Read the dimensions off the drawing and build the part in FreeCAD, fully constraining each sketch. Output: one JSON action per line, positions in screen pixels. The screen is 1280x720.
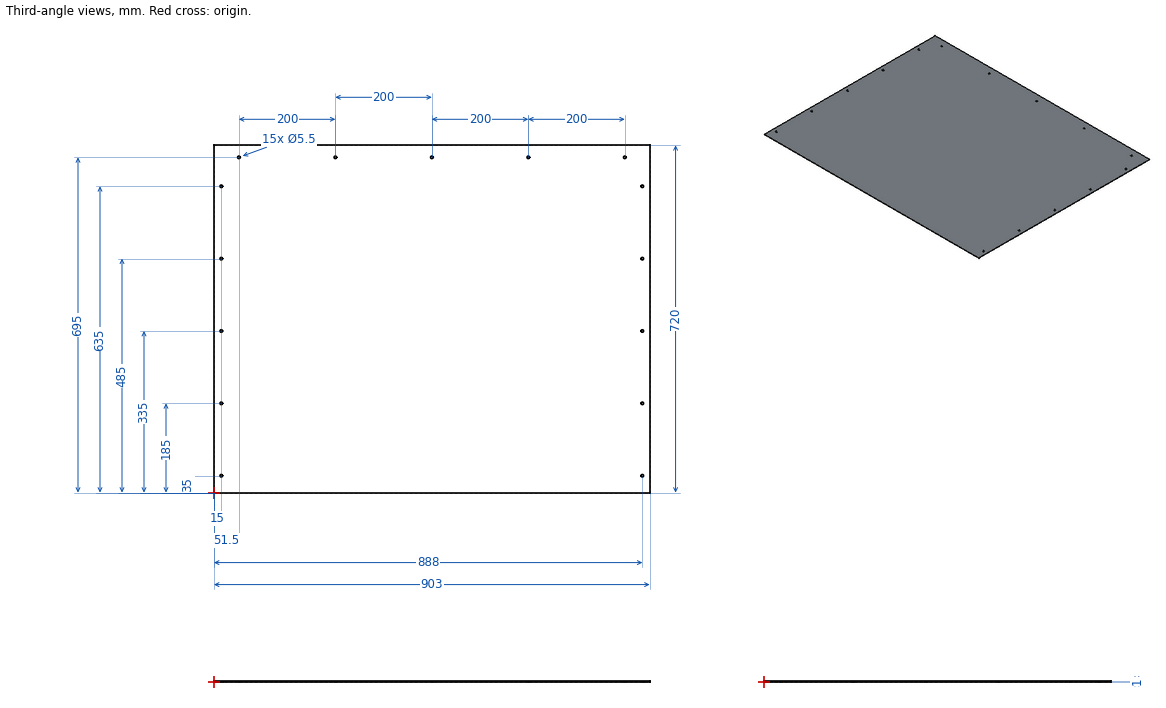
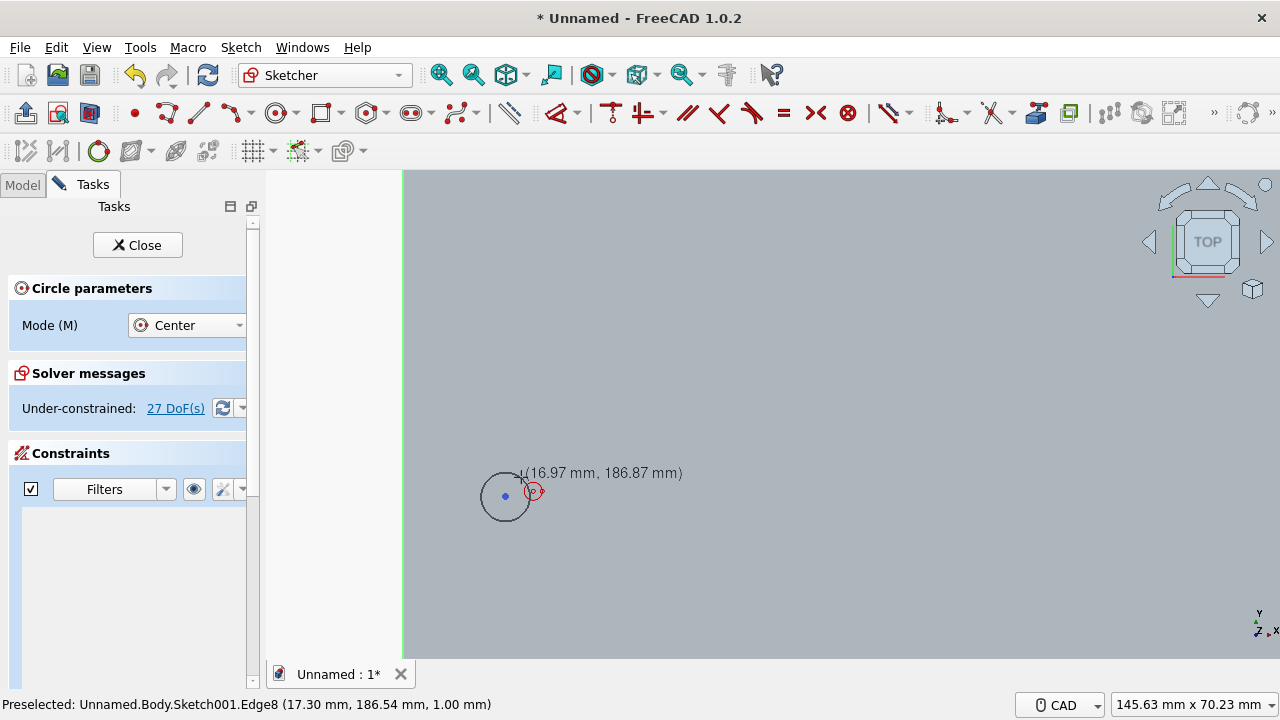
{"action": "scroll", "coordinate": [523, 483], "scroll_direction": "down", "scroll_amount": 14}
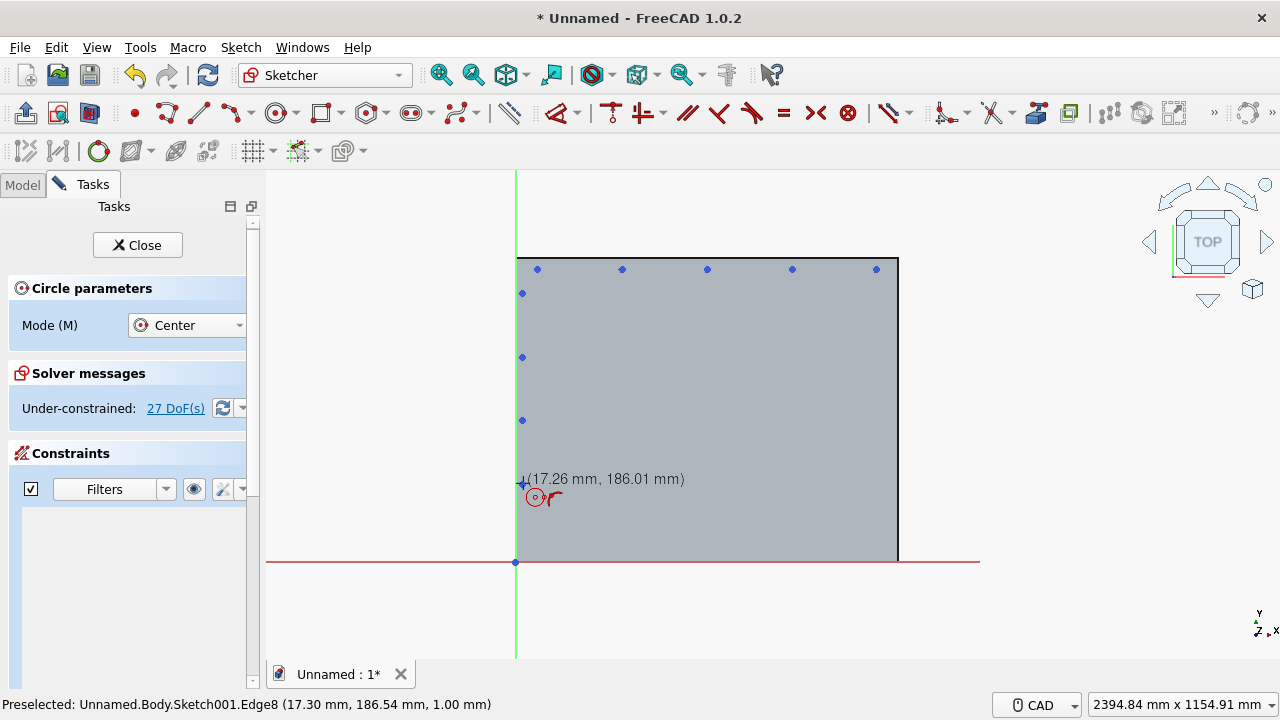
{"action": "scroll", "coordinate": [522, 548], "scroll_direction": "up", "scroll_amount": 15}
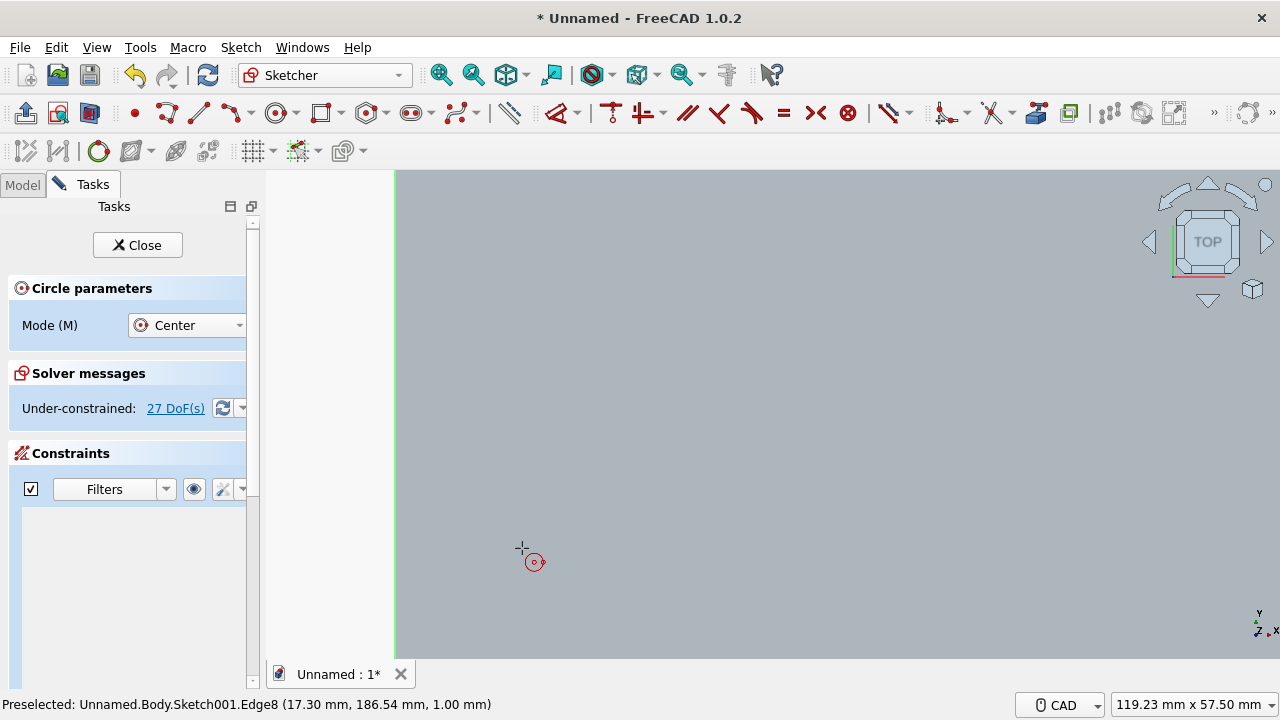
{"action": "scroll", "coordinate": [522, 549], "scroll_direction": "down", "scroll_amount": 15}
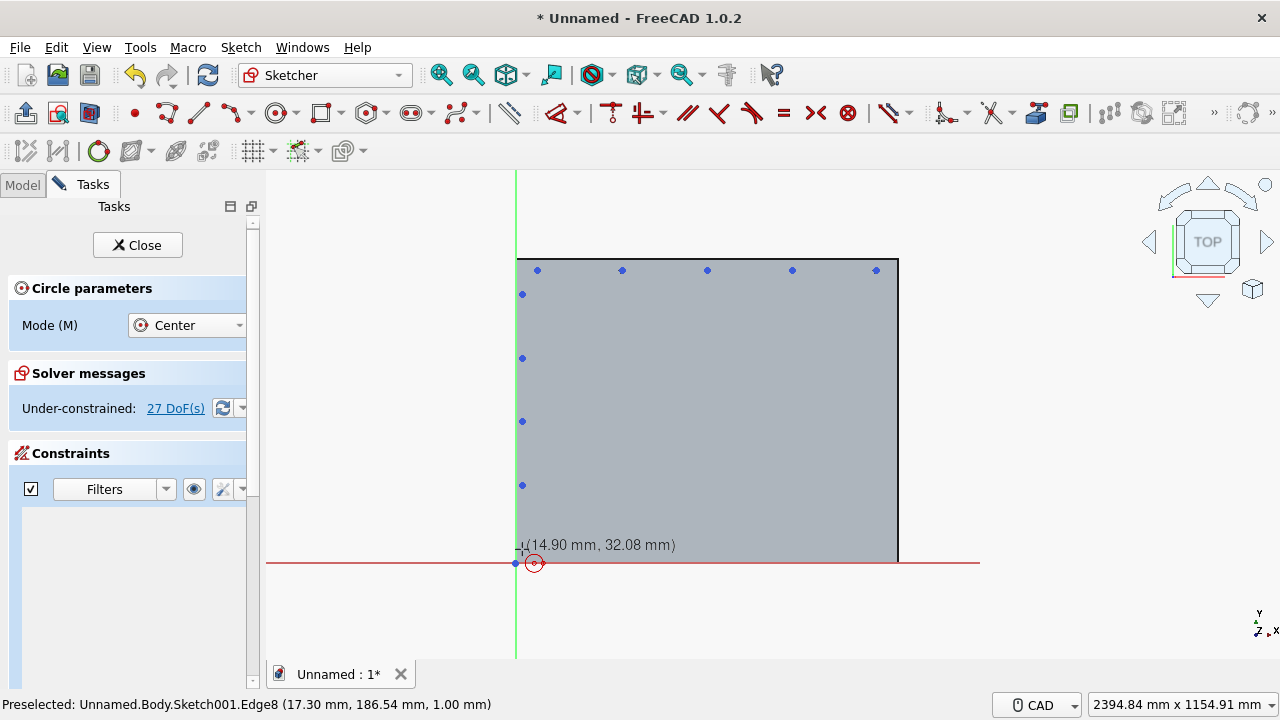
{"action": "scroll", "coordinate": [522, 549], "scroll_direction": "up", "scroll_amount": 5}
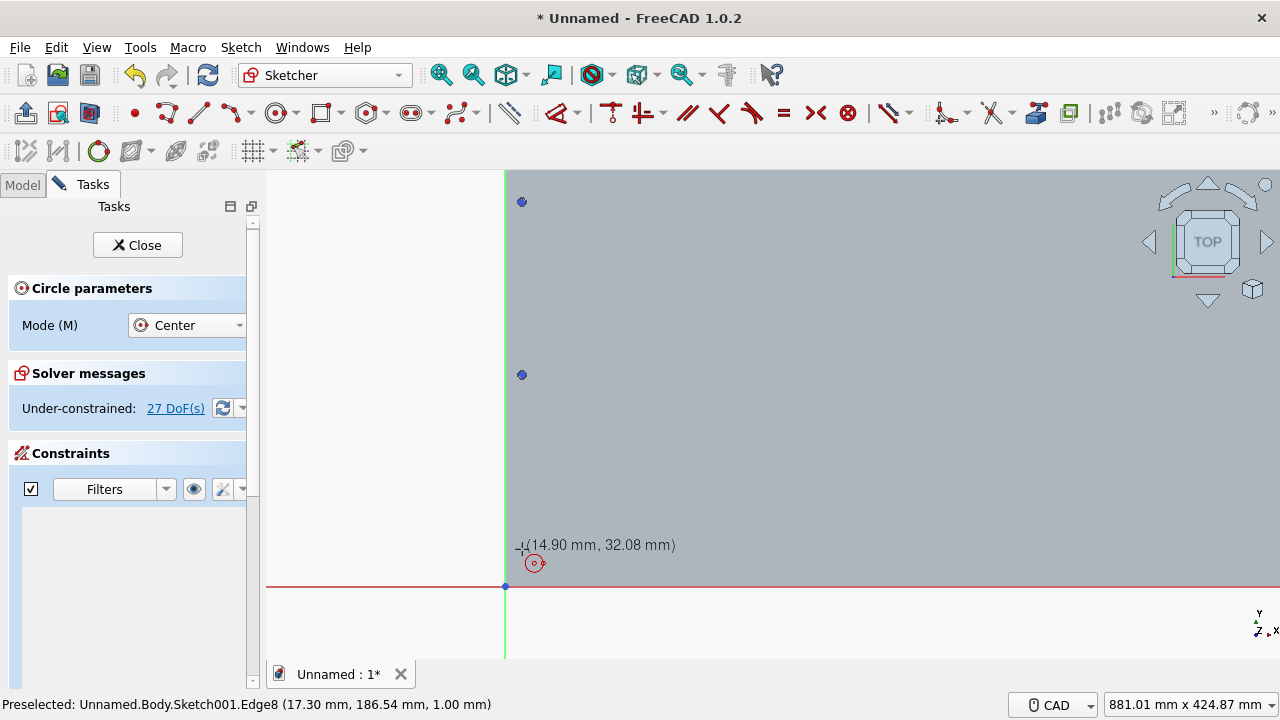
{"action": "left_click", "coordinate": [522, 546]}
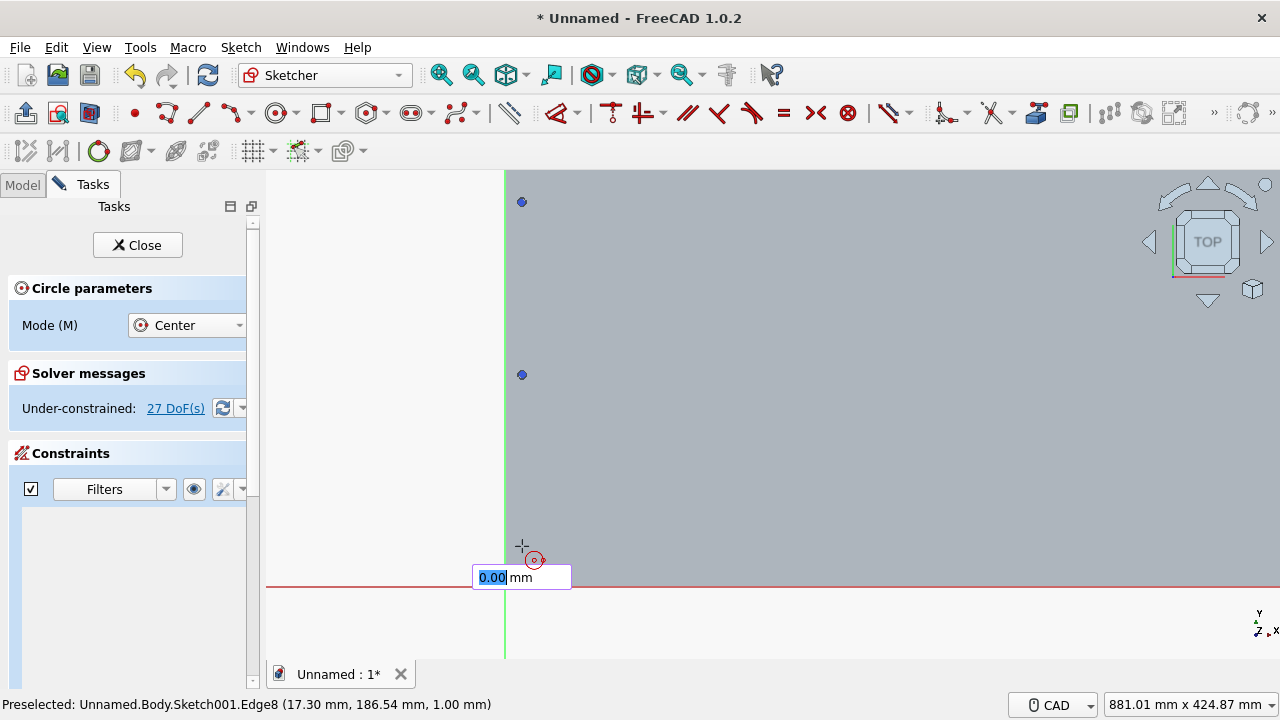
{"action": "scroll", "coordinate": [525, 544], "scroll_direction": "up", "scroll_amount": 9}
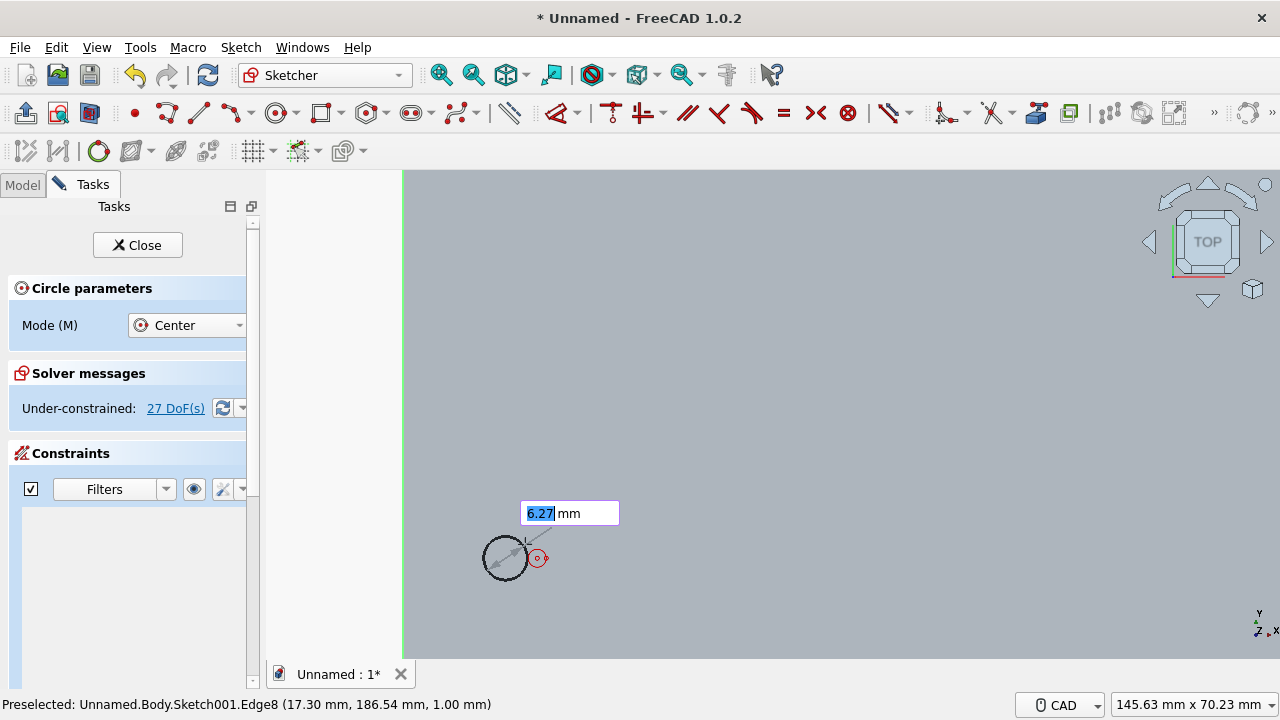
{"action": "left_click", "coordinate": [521, 541]}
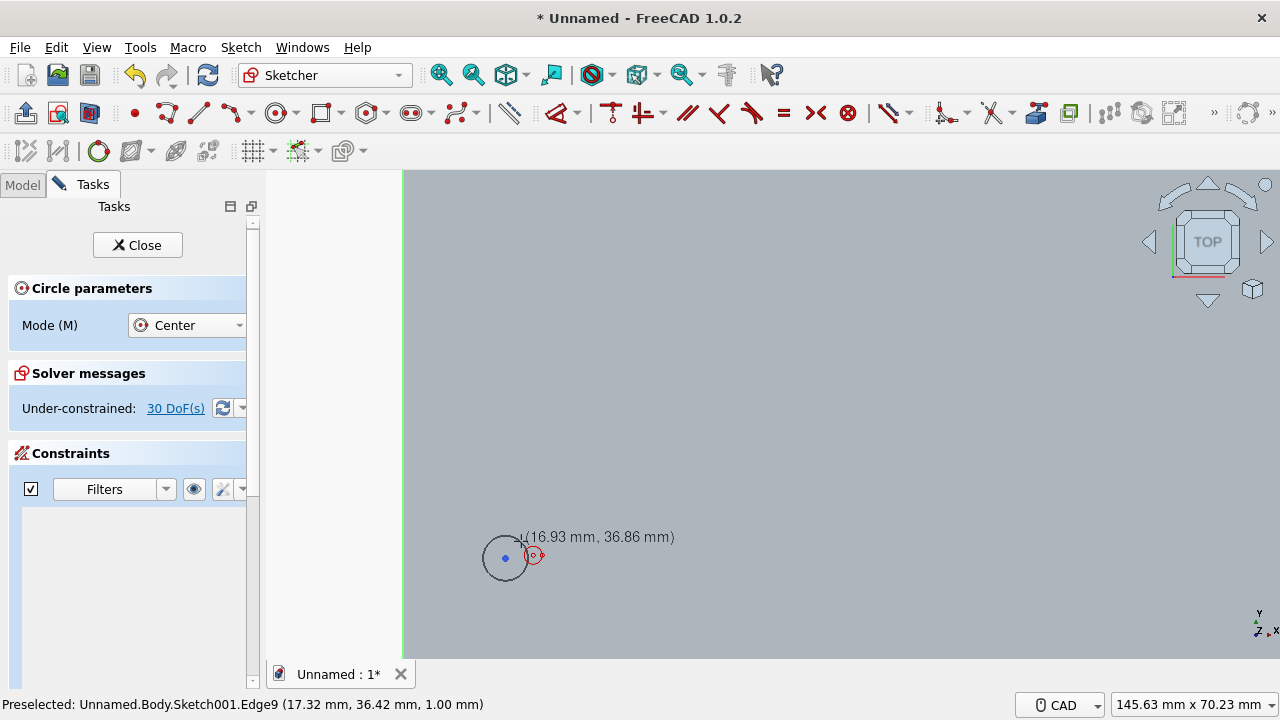
{"action": "scroll", "coordinate": [523, 547], "scroll_direction": "down", "scroll_amount": 14}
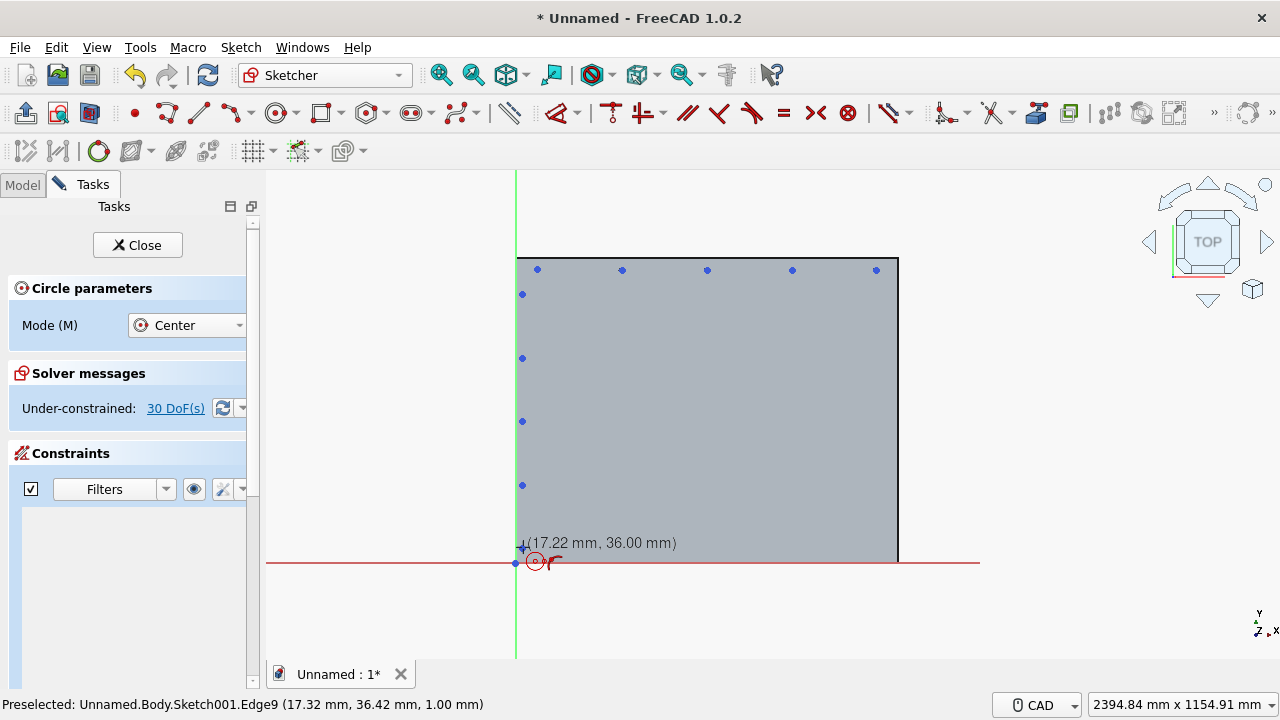
{"action": "scroll", "coordinate": [892, 548], "scroll_direction": "up", "scroll_amount": 15}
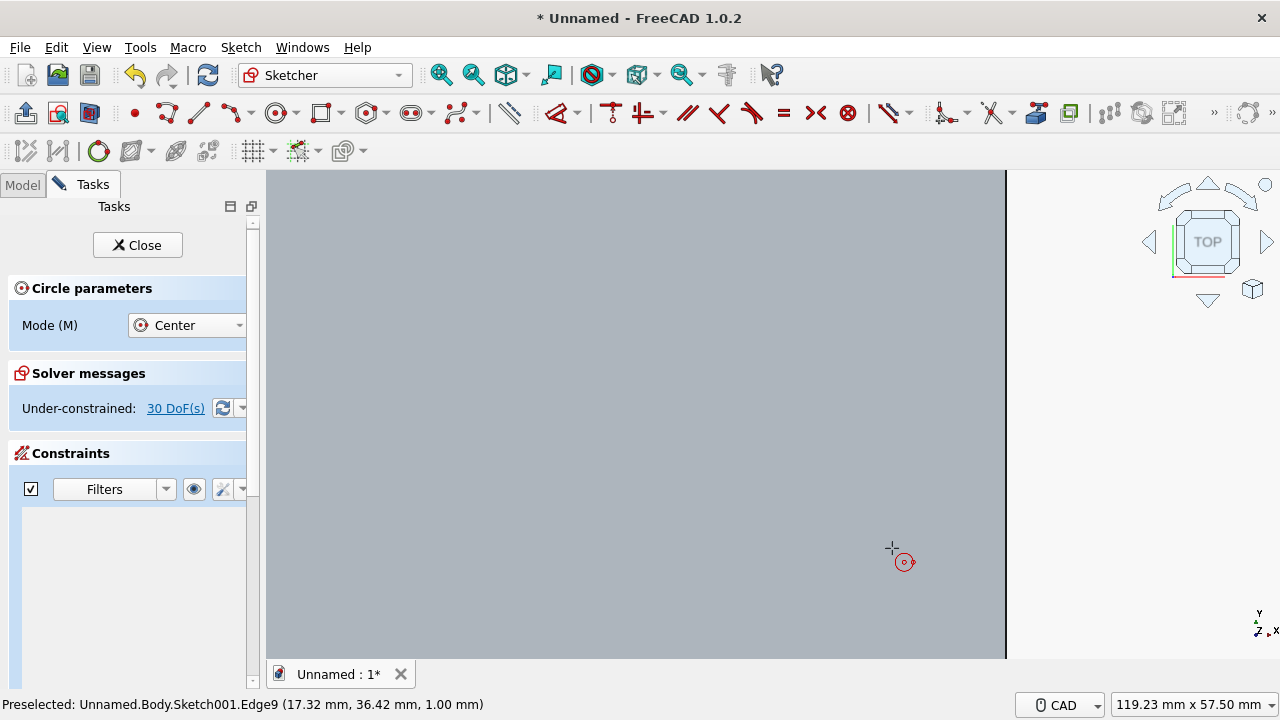
{"action": "scroll", "coordinate": [893, 548], "scroll_direction": "down", "scroll_amount": 15}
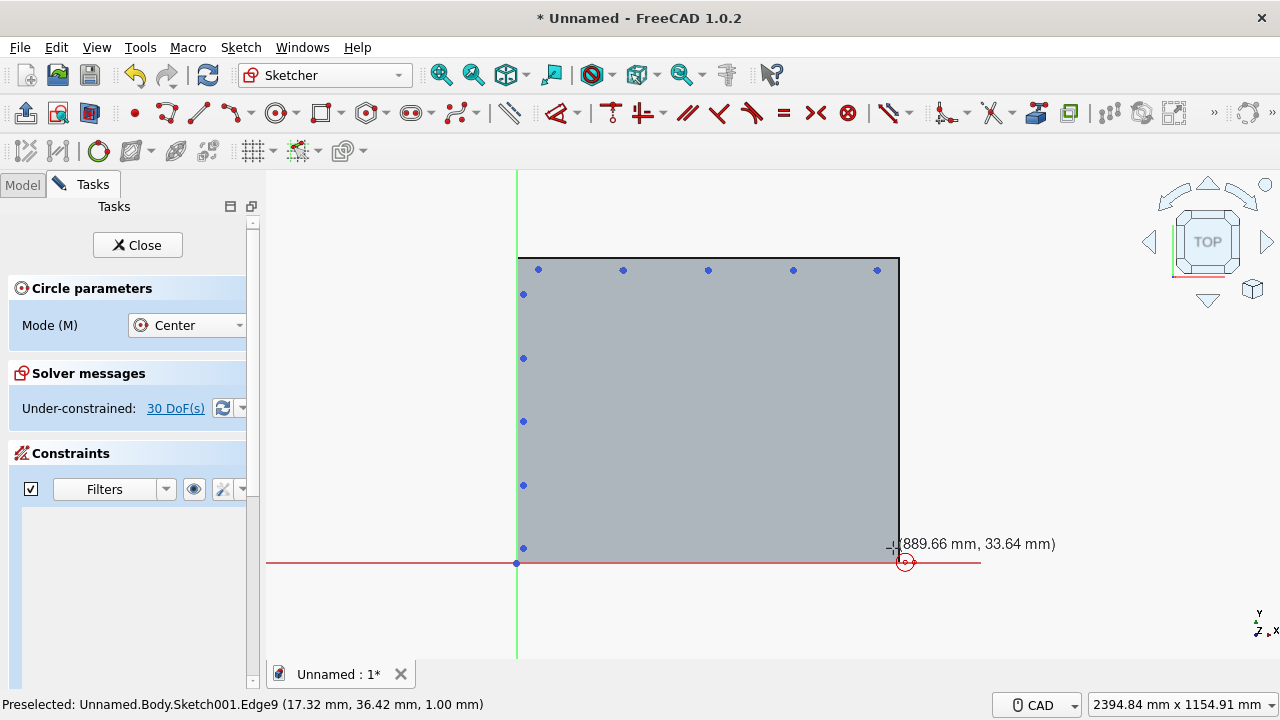
{"action": "left_click", "coordinate": [893, 548]}